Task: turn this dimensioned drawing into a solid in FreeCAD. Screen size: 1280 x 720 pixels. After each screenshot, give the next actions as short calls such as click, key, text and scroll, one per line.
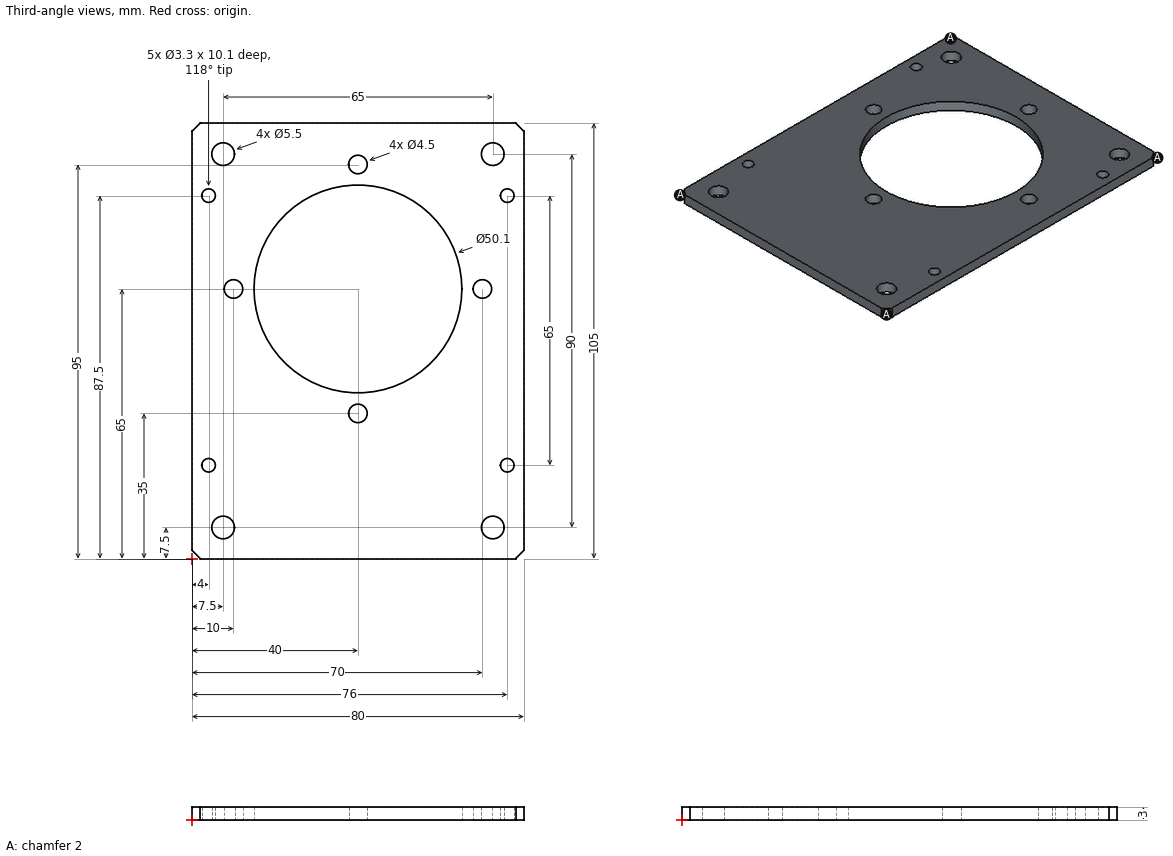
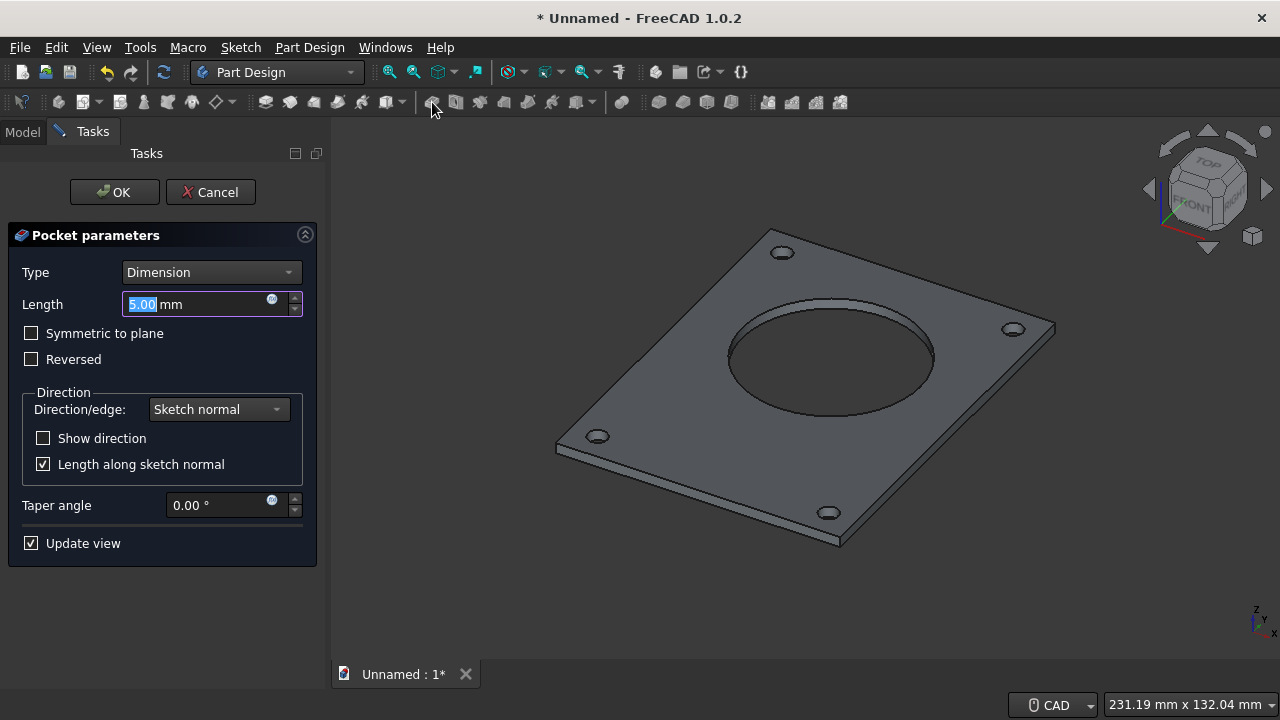
click(212, 272)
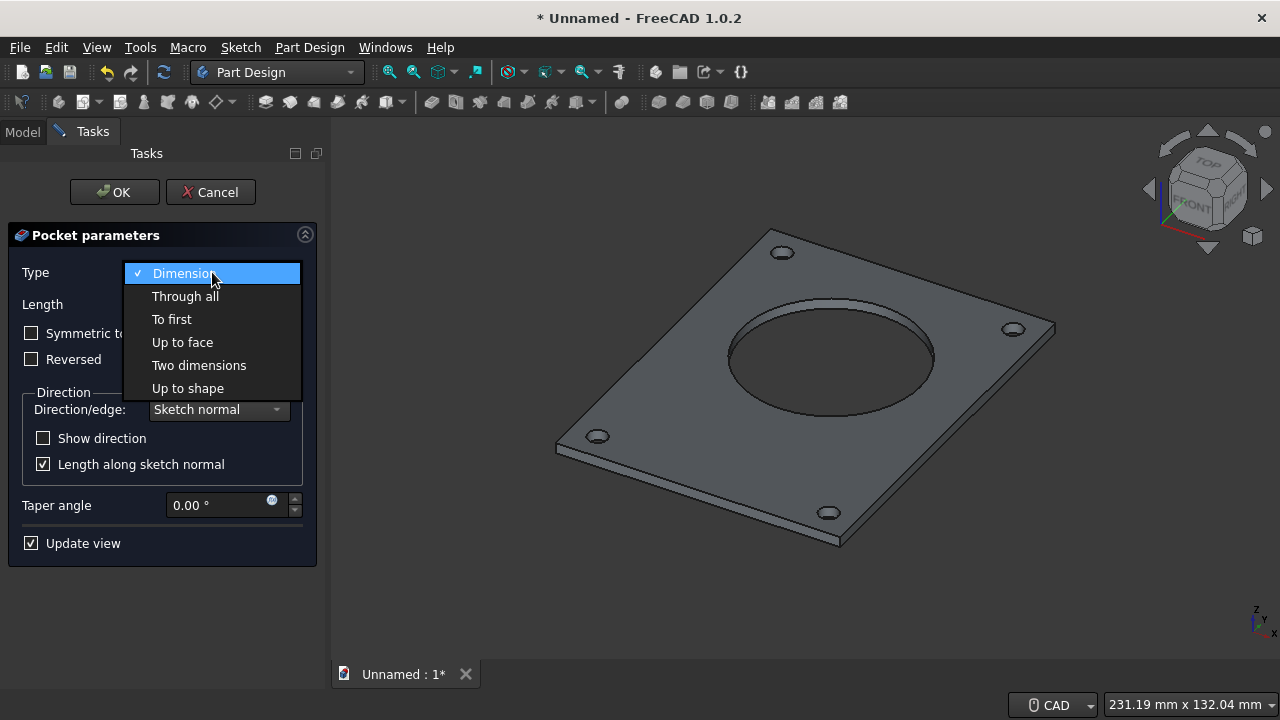
click(212, 296)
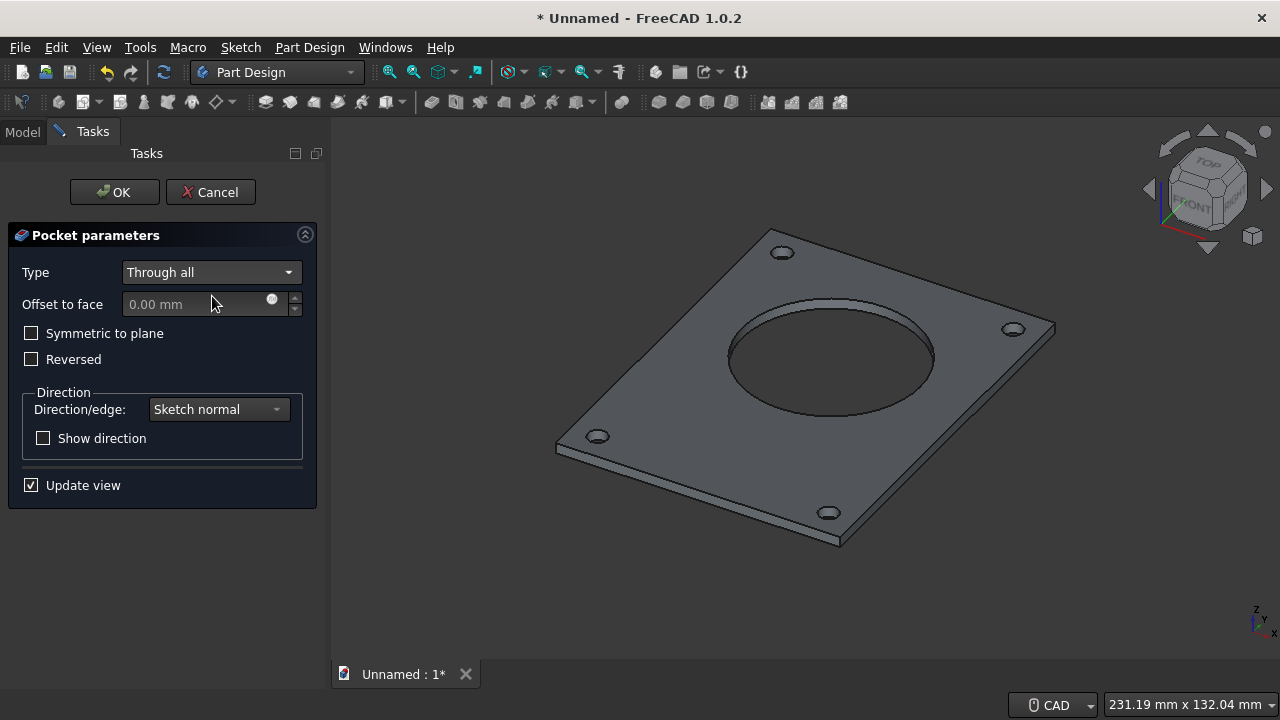
click(115, 192)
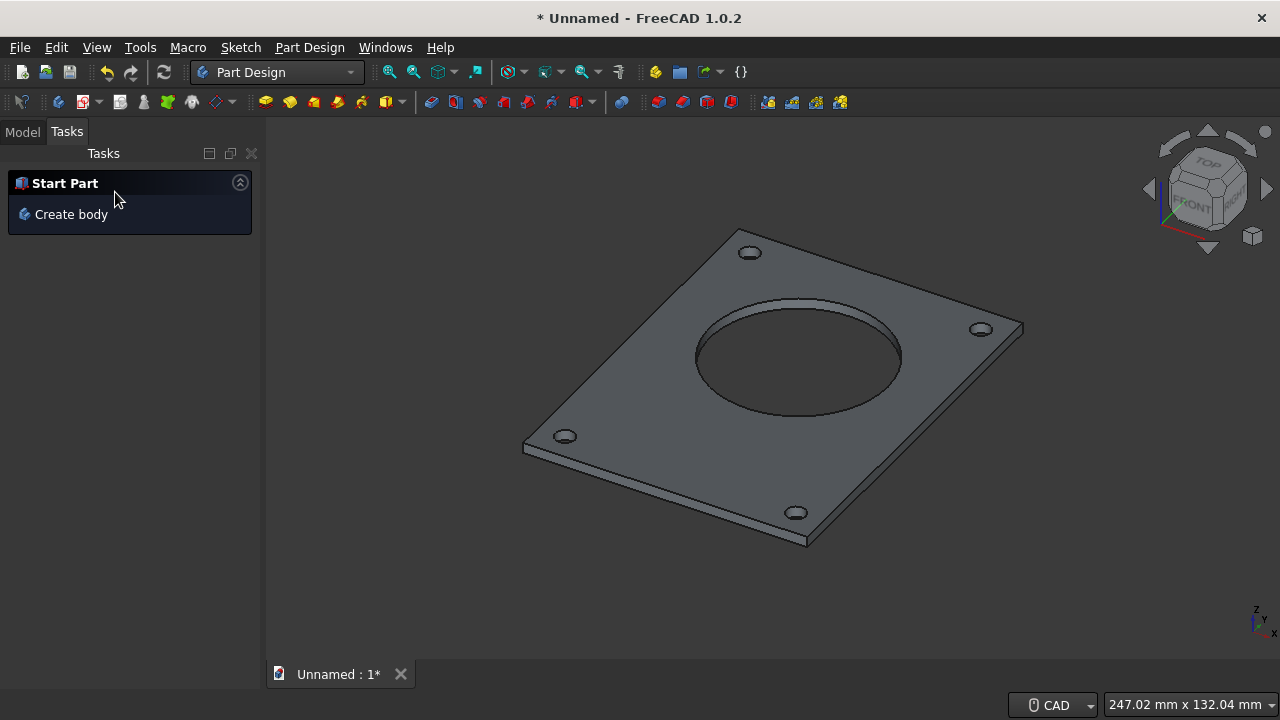
click(752, 457)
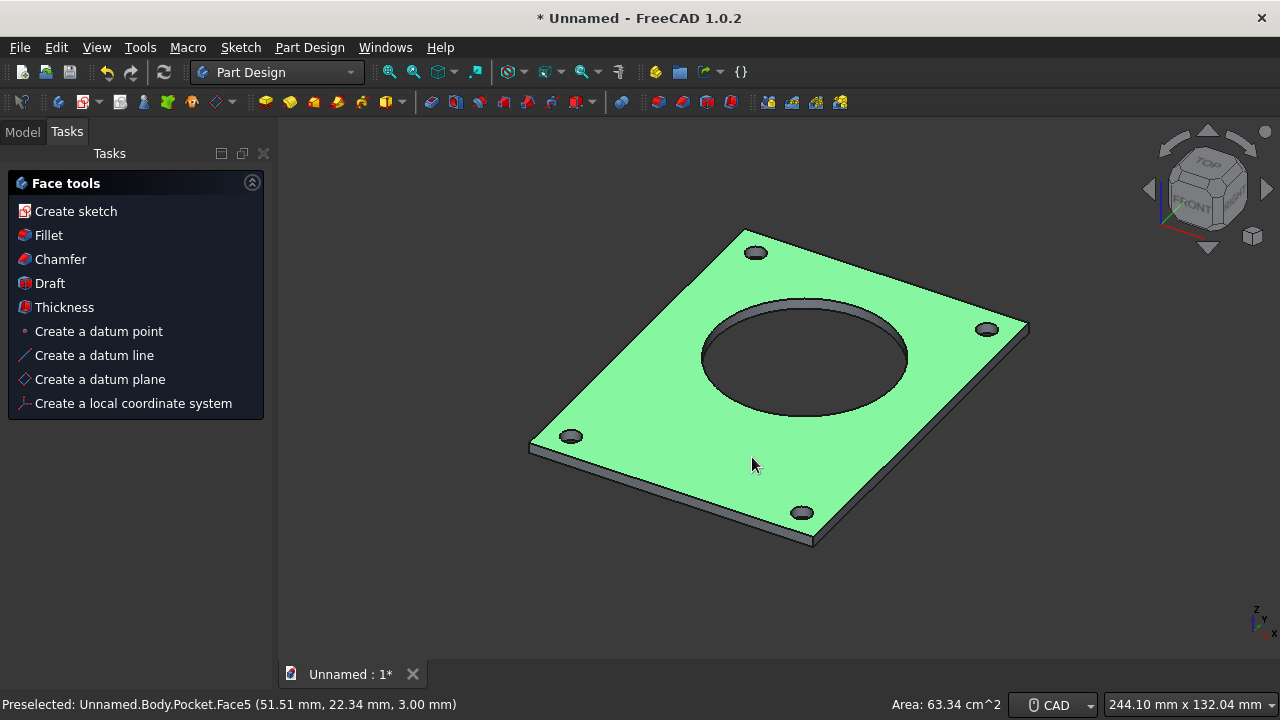
click(84, 102)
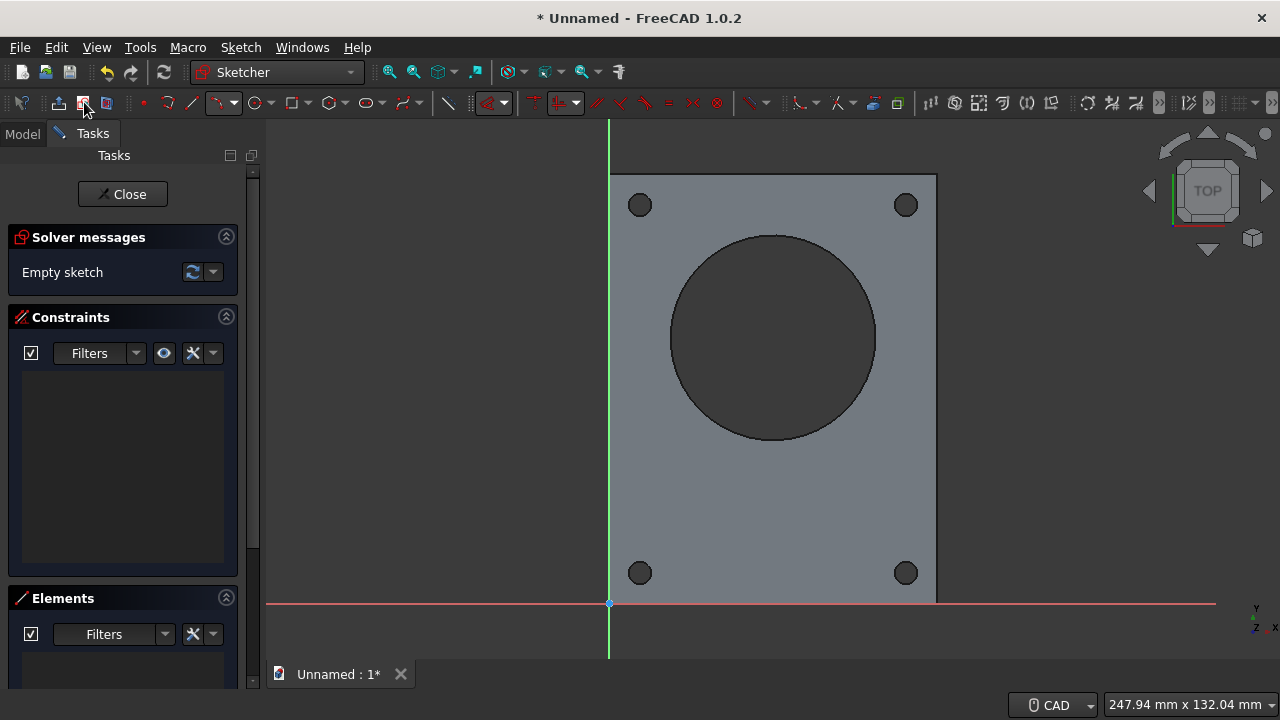
click(256, 104)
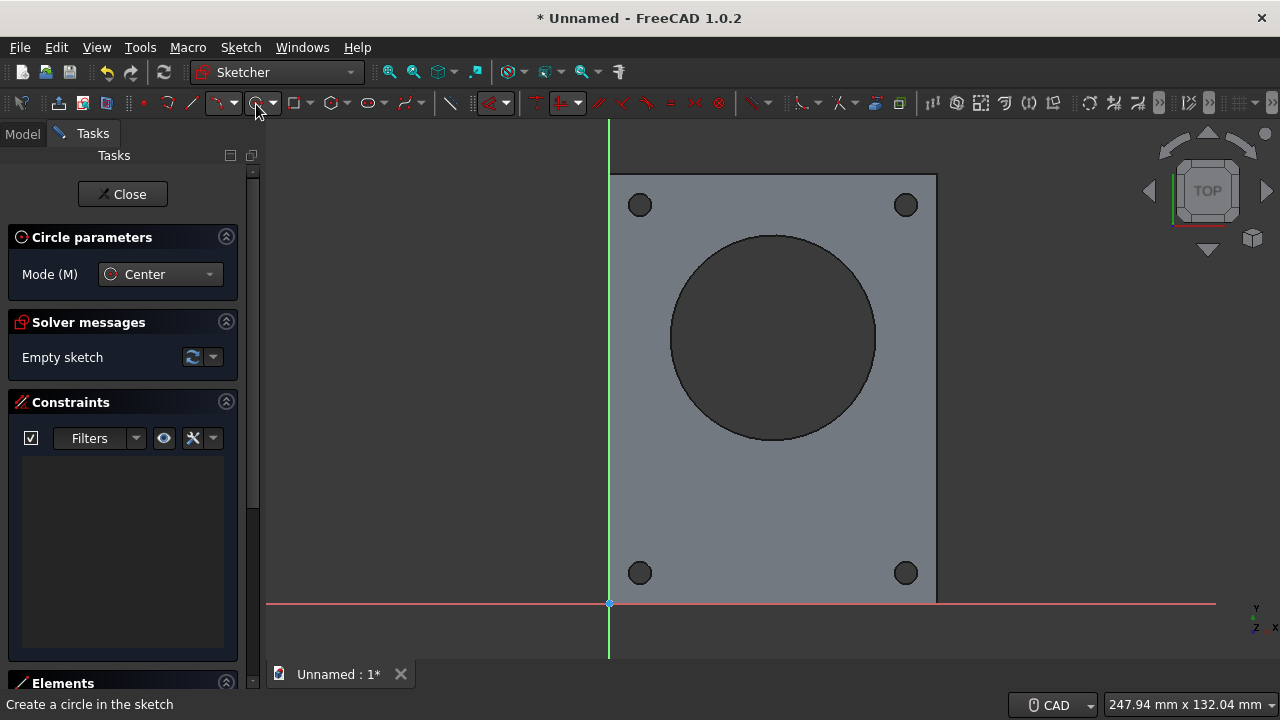
scroll(773, 215, up, 5)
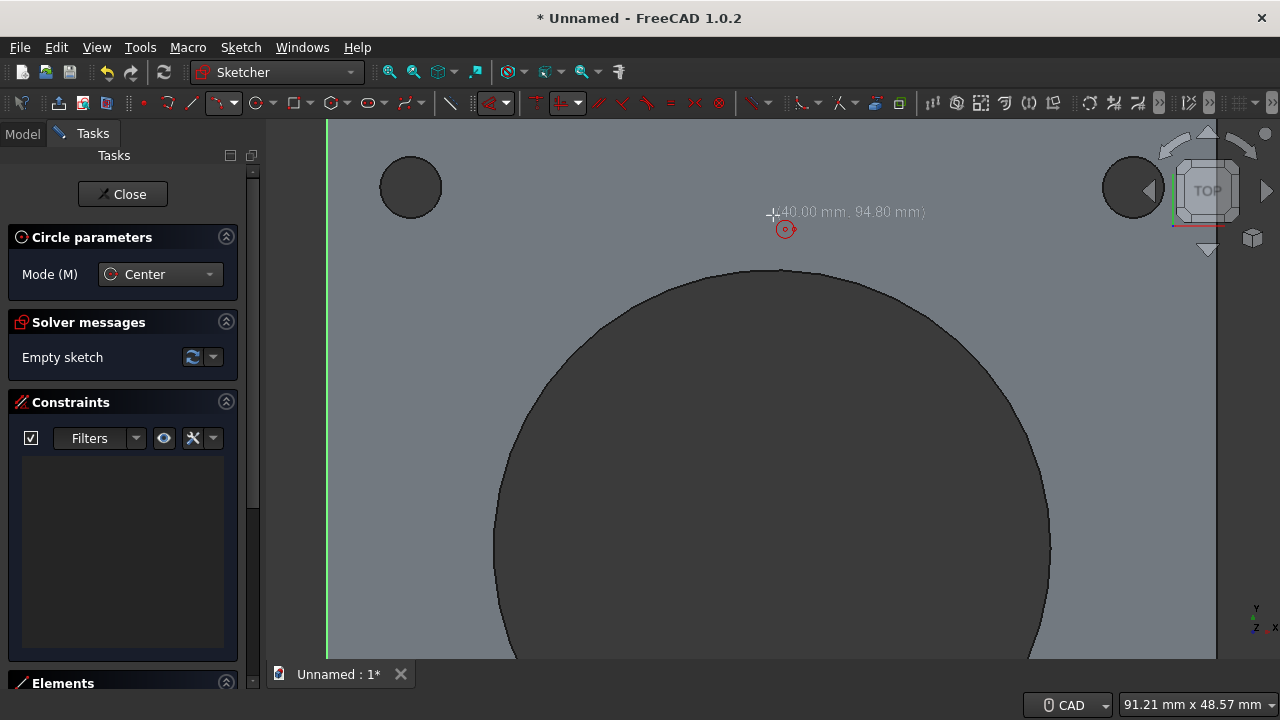
click(772, 215)
move(790, 198)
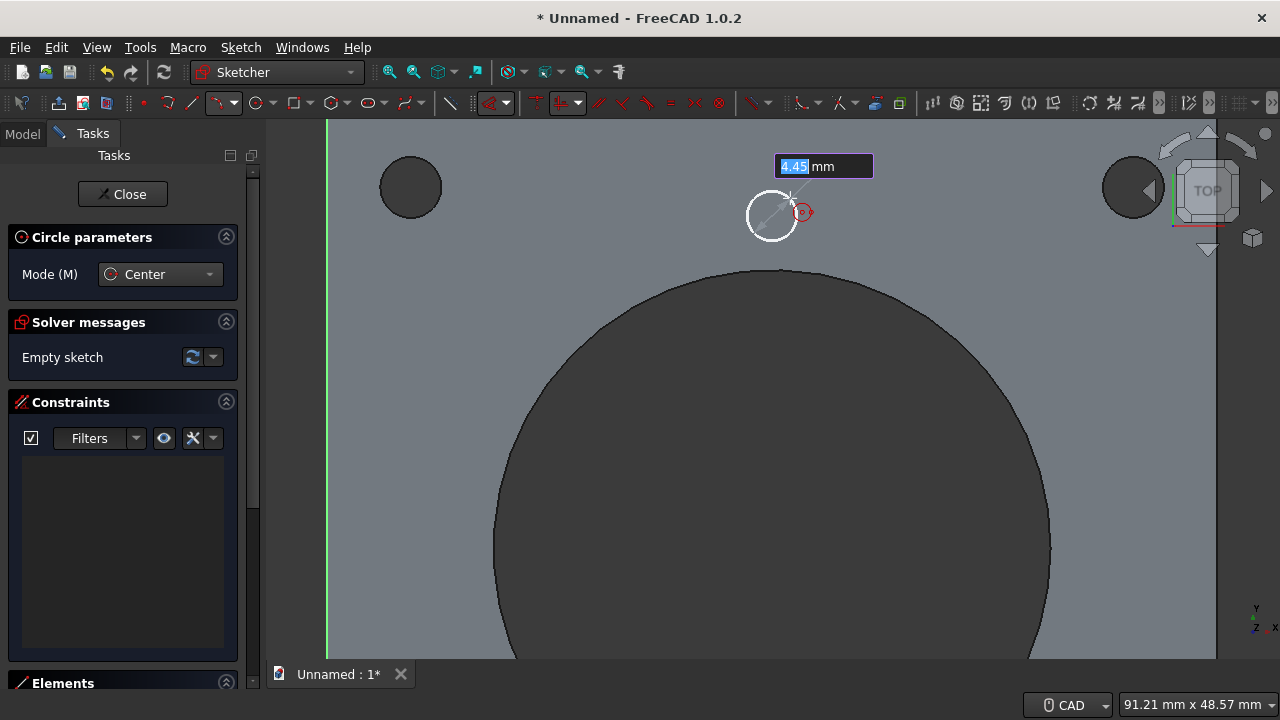
text(4.5)
key(Return)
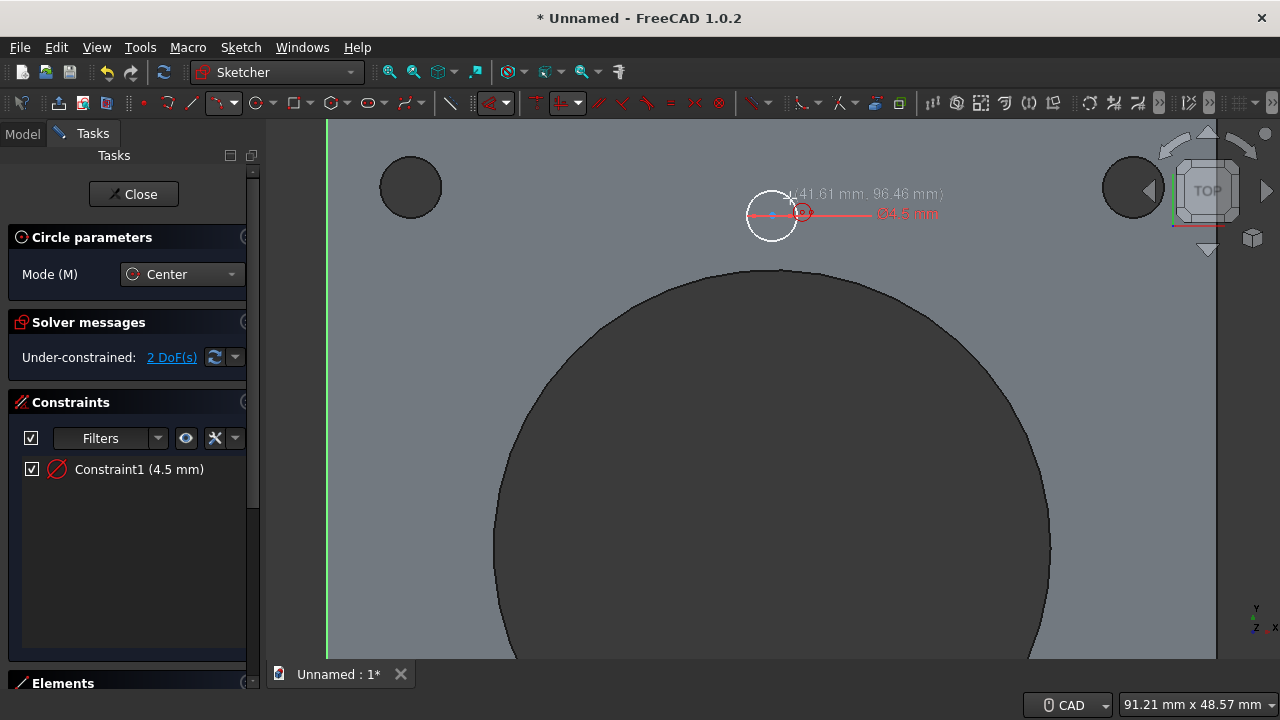
click(439, 549)
move(456, 531)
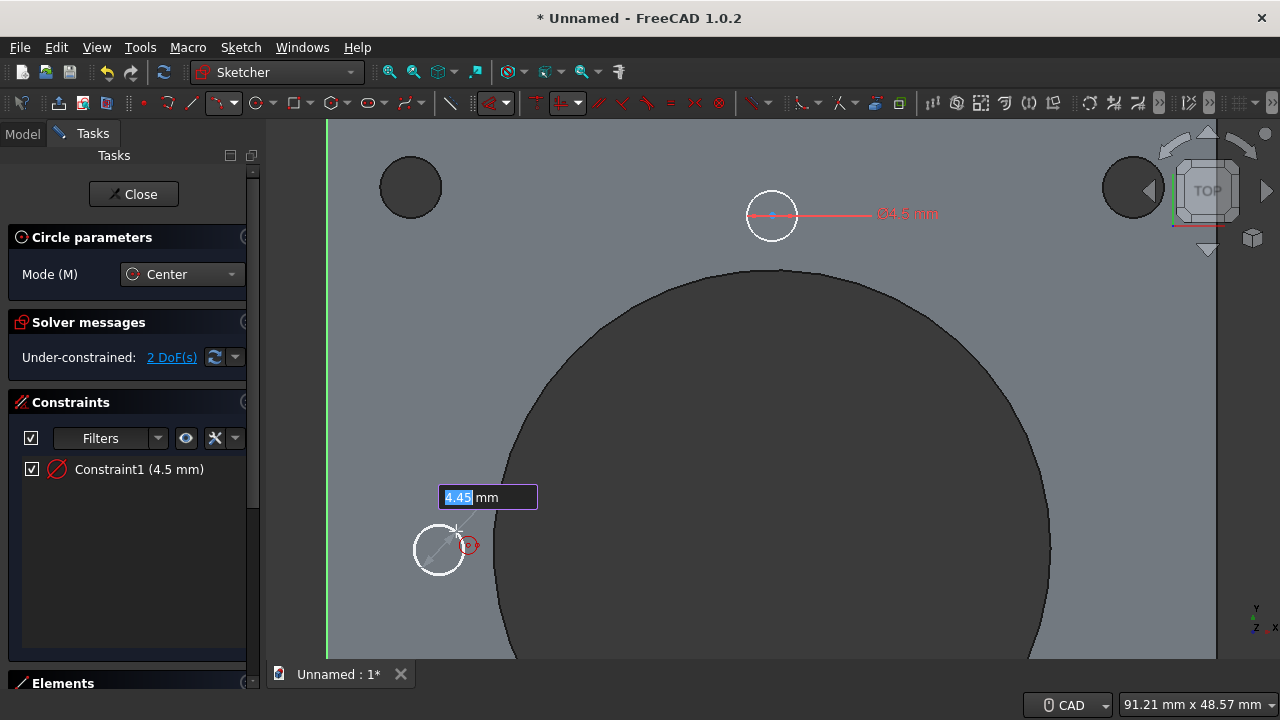
text(4.5)
key(Return)